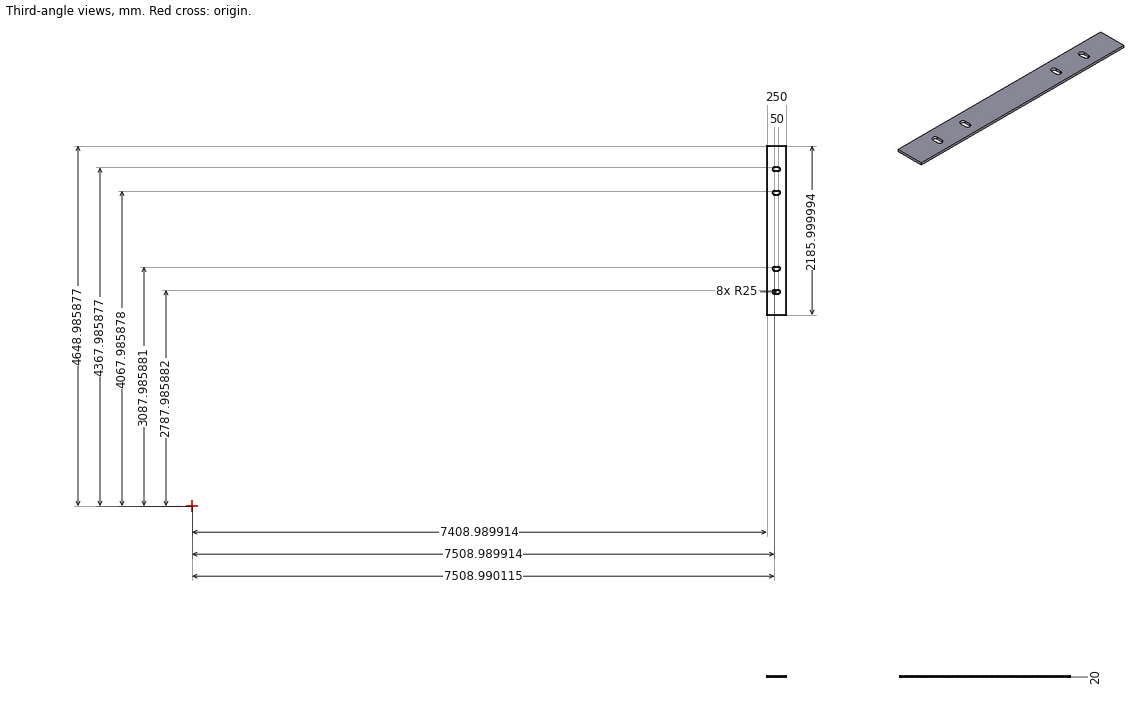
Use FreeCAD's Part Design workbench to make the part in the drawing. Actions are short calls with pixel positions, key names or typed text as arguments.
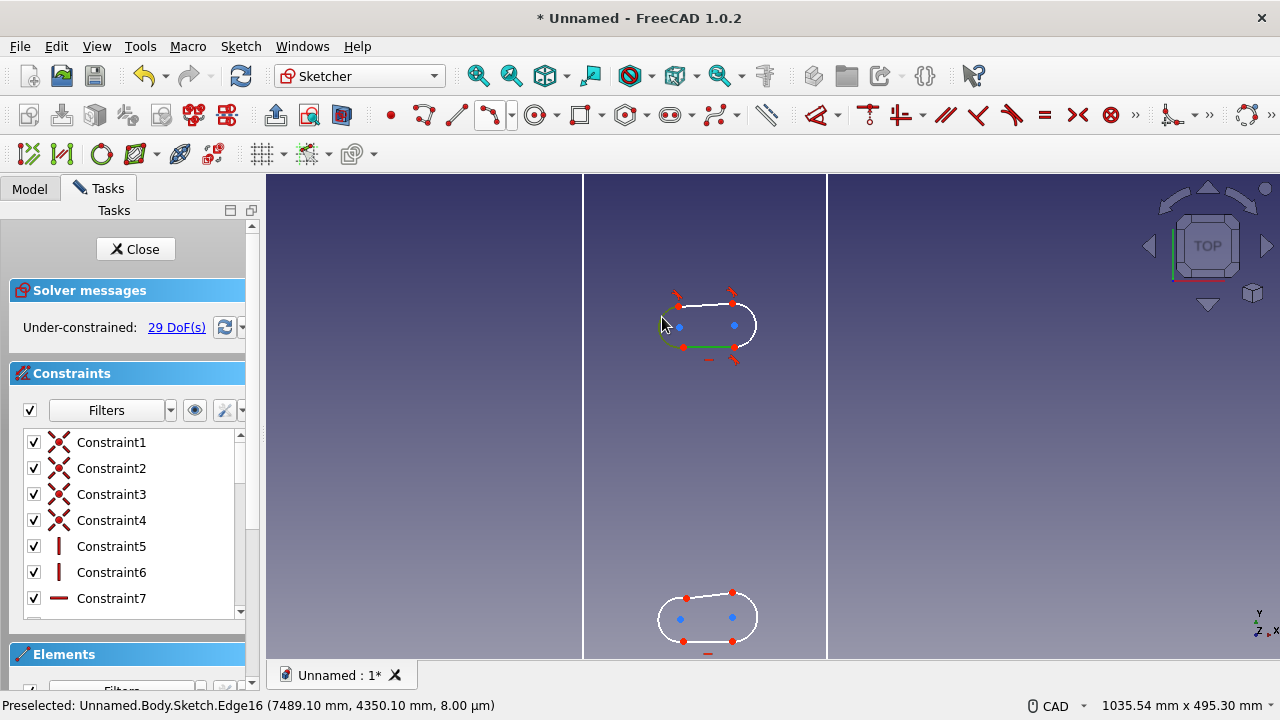
key(t)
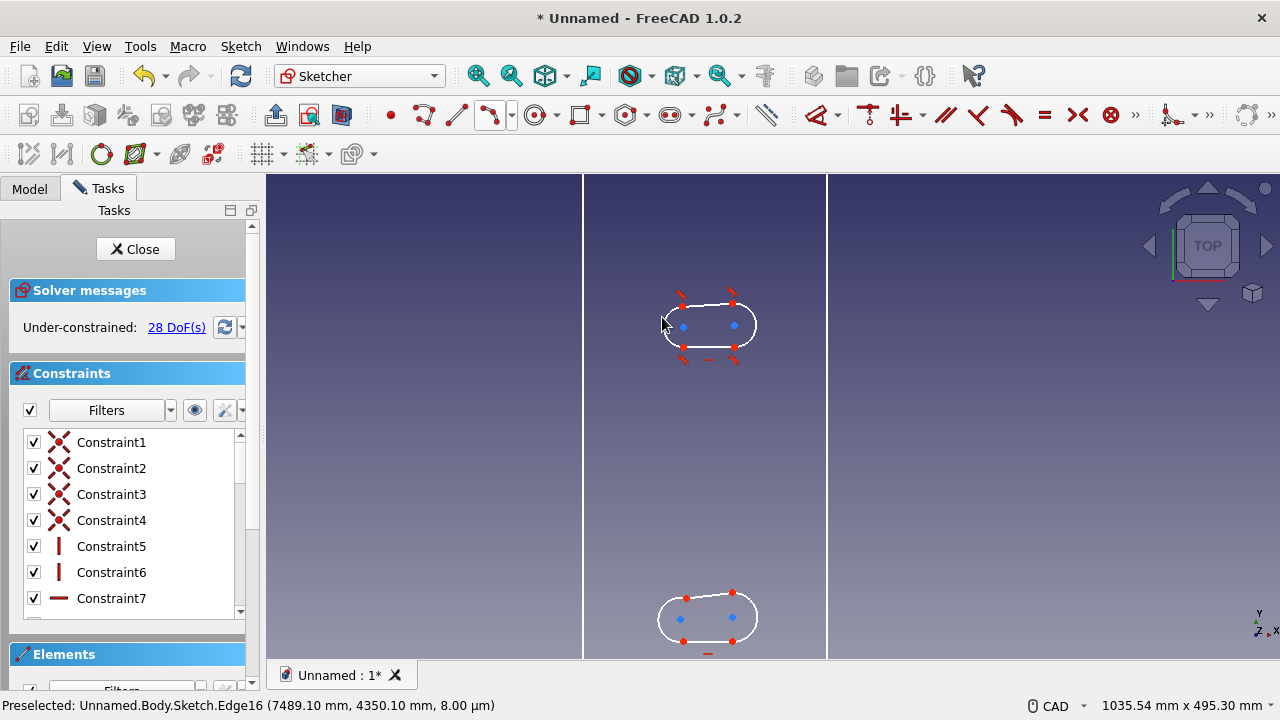
click(700, 597)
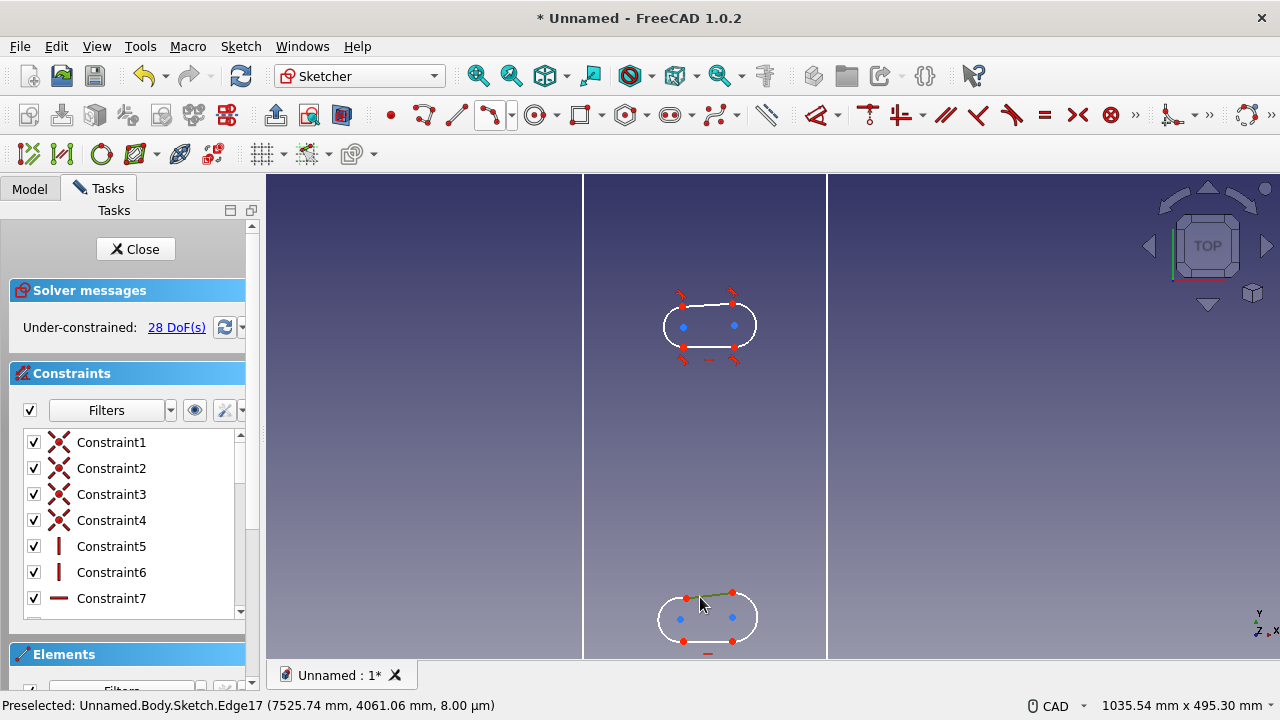
click(753, 603)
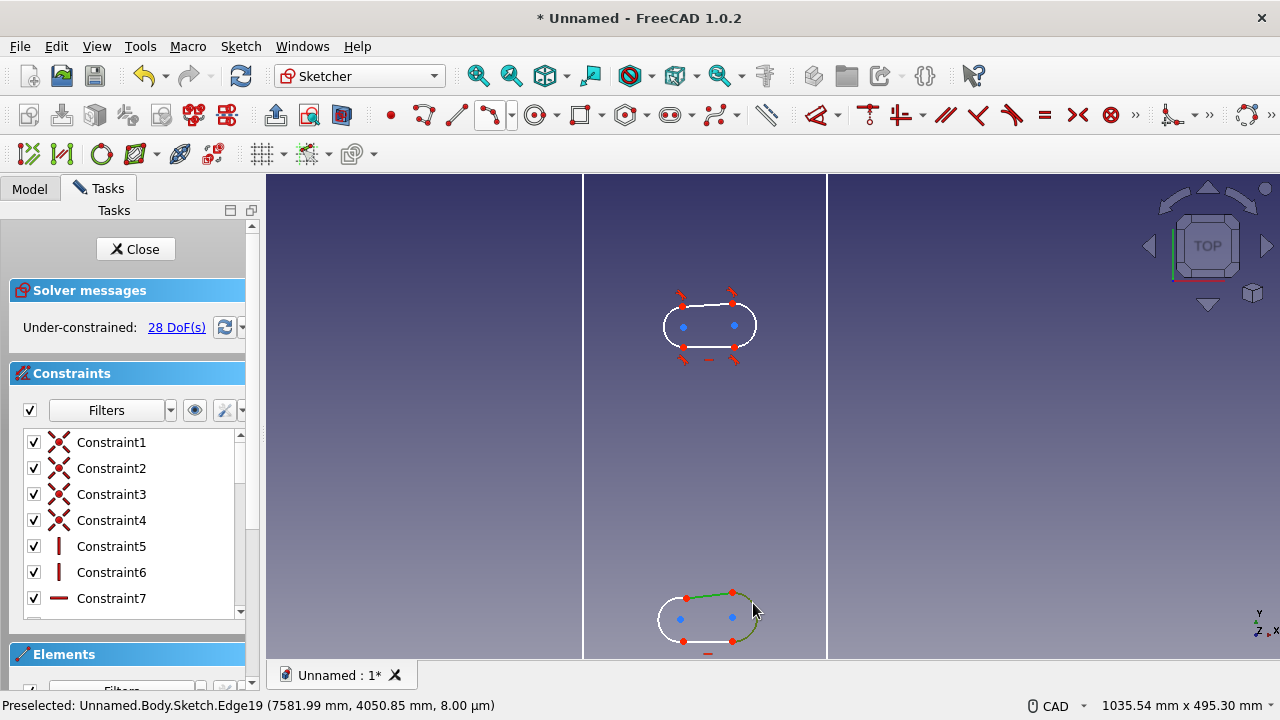
key(t)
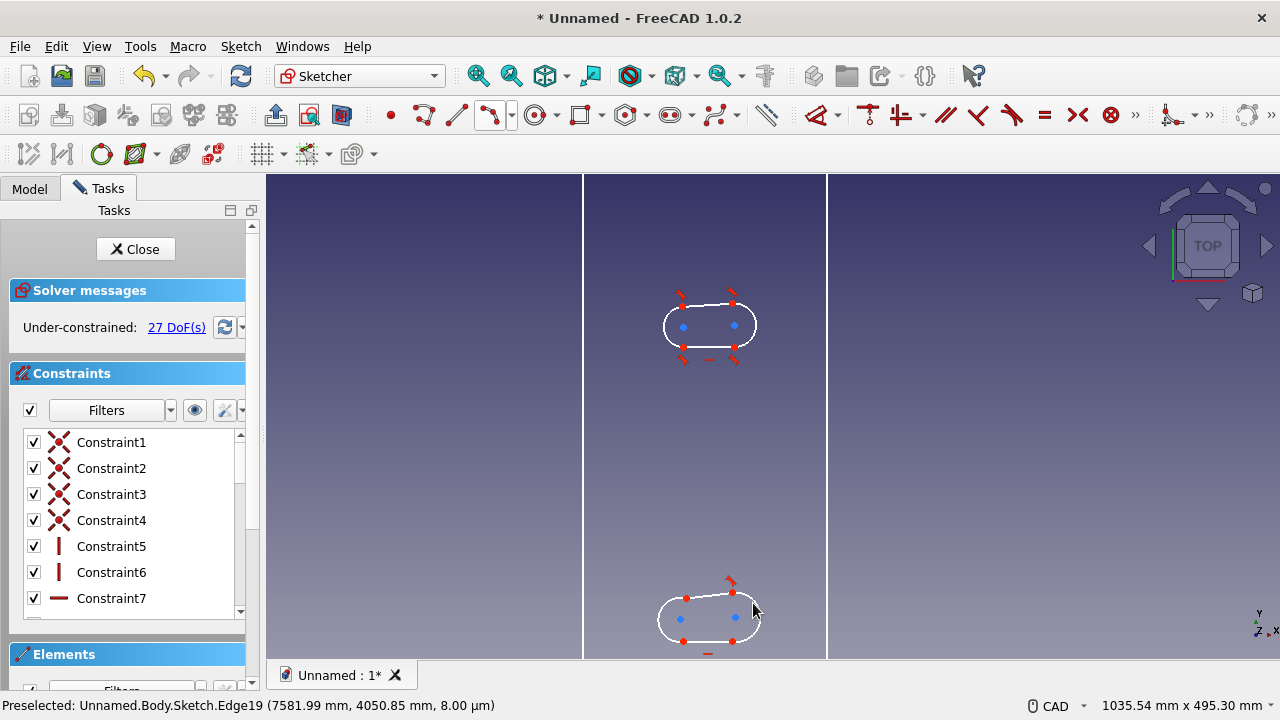
click(700, 597)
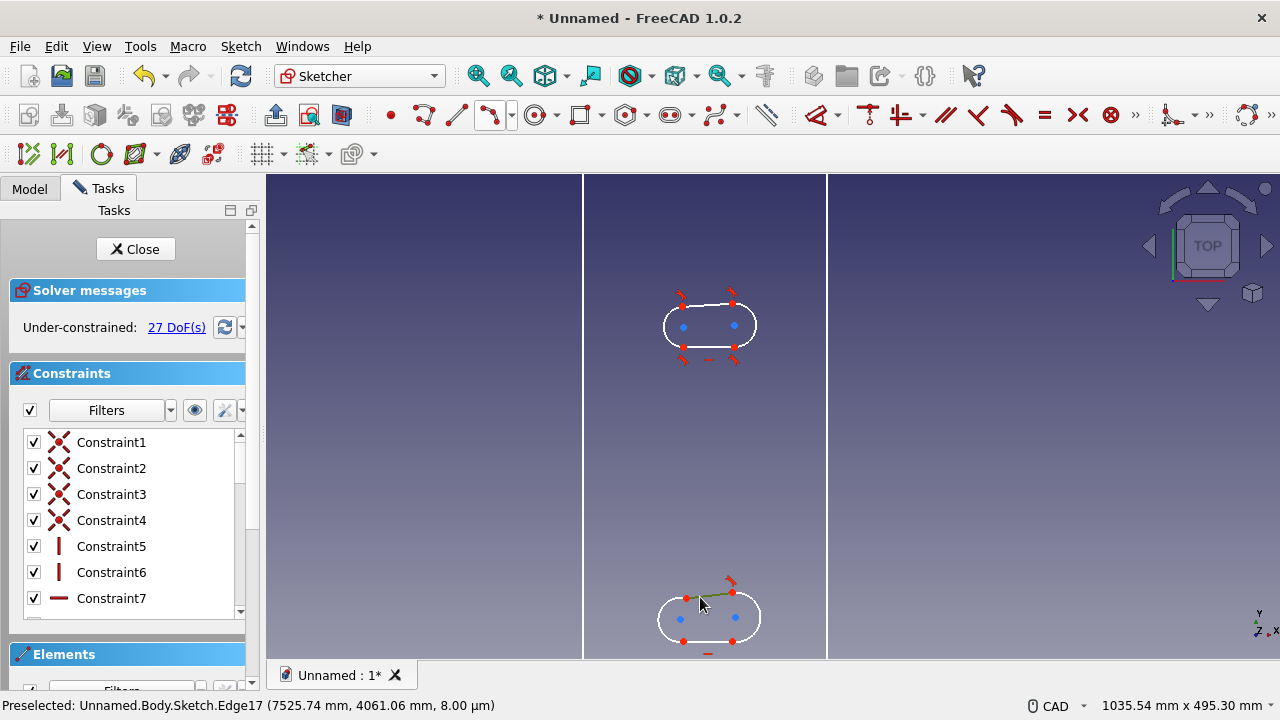
click(665, 604)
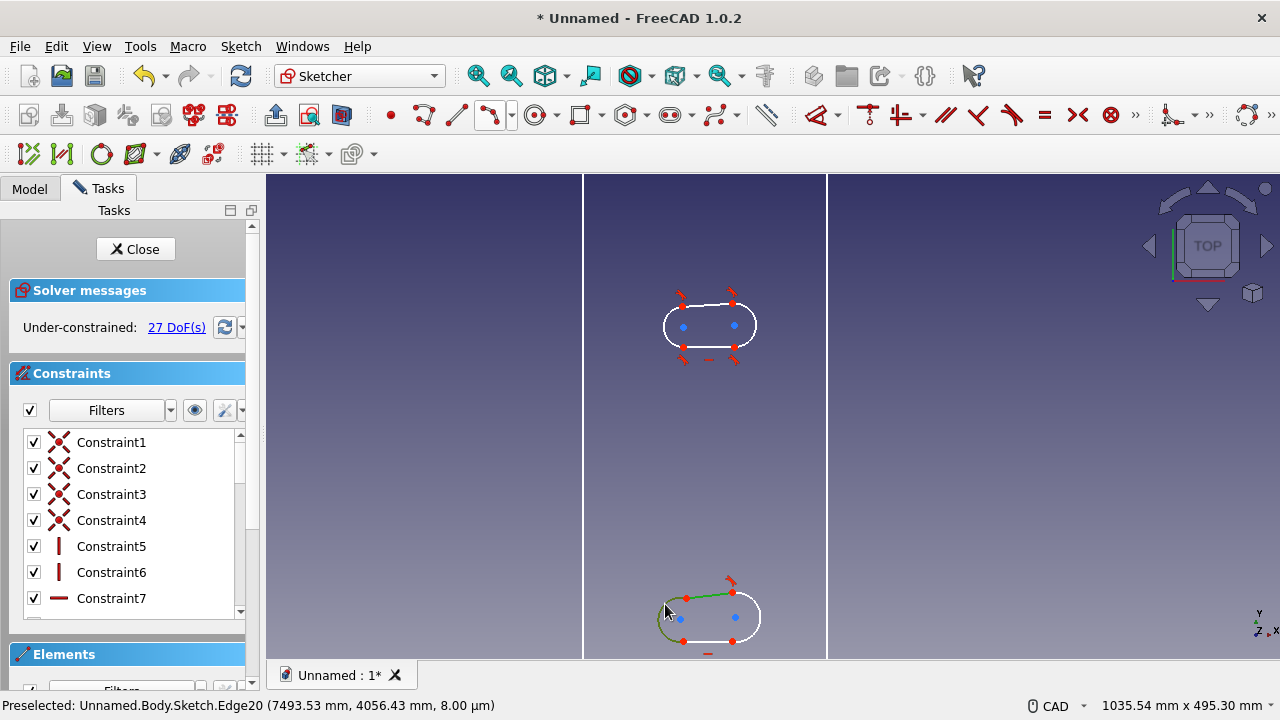
click(1012, 116)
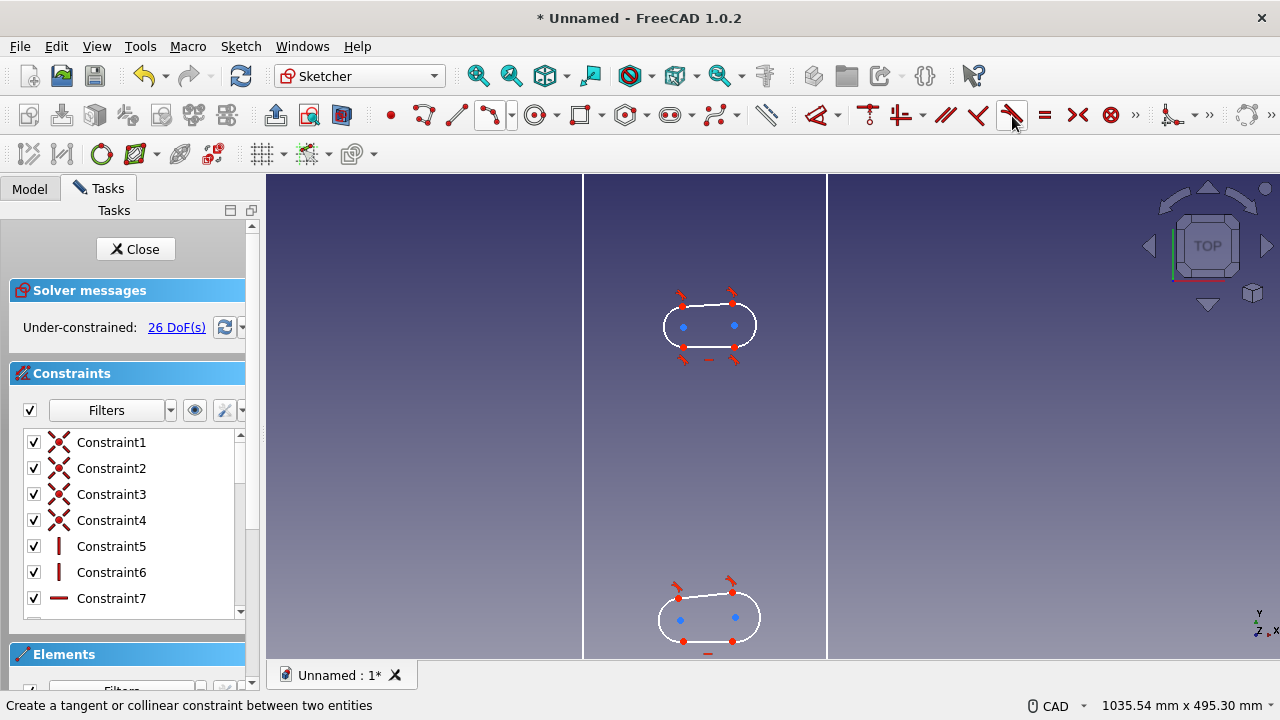
scroll(704, 311, down, 10)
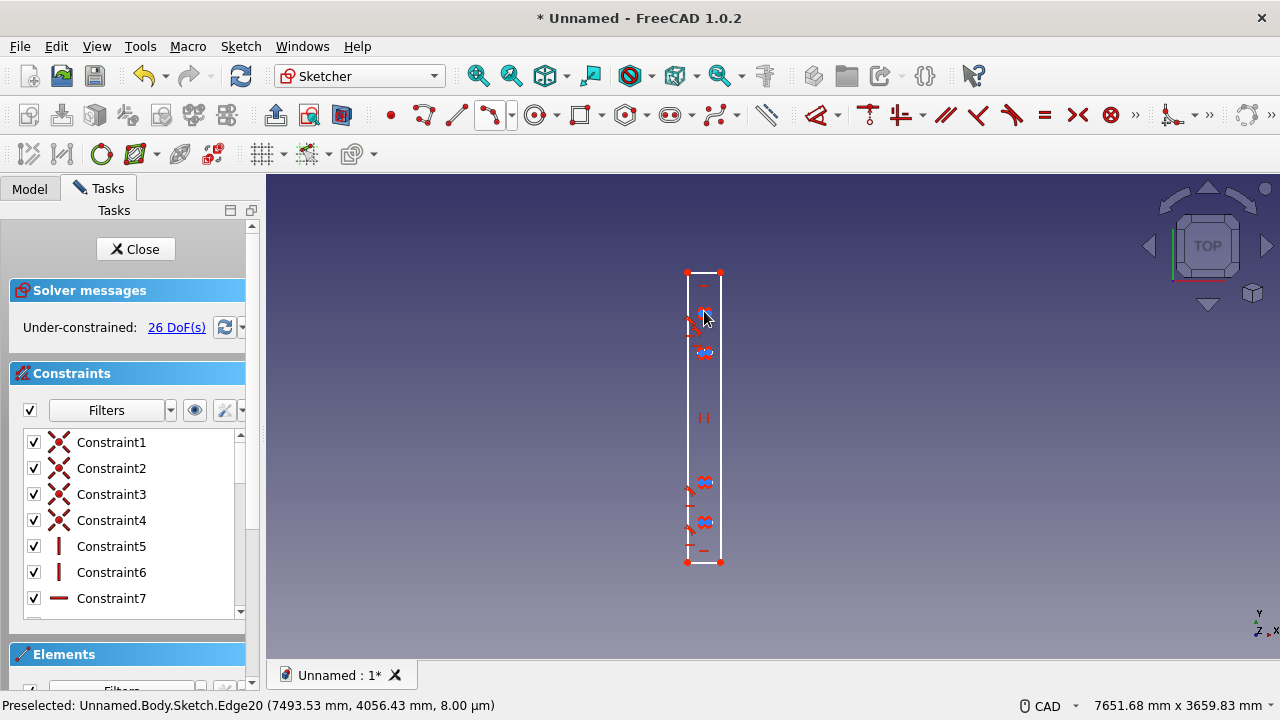
scroll(706, 356, up, 10)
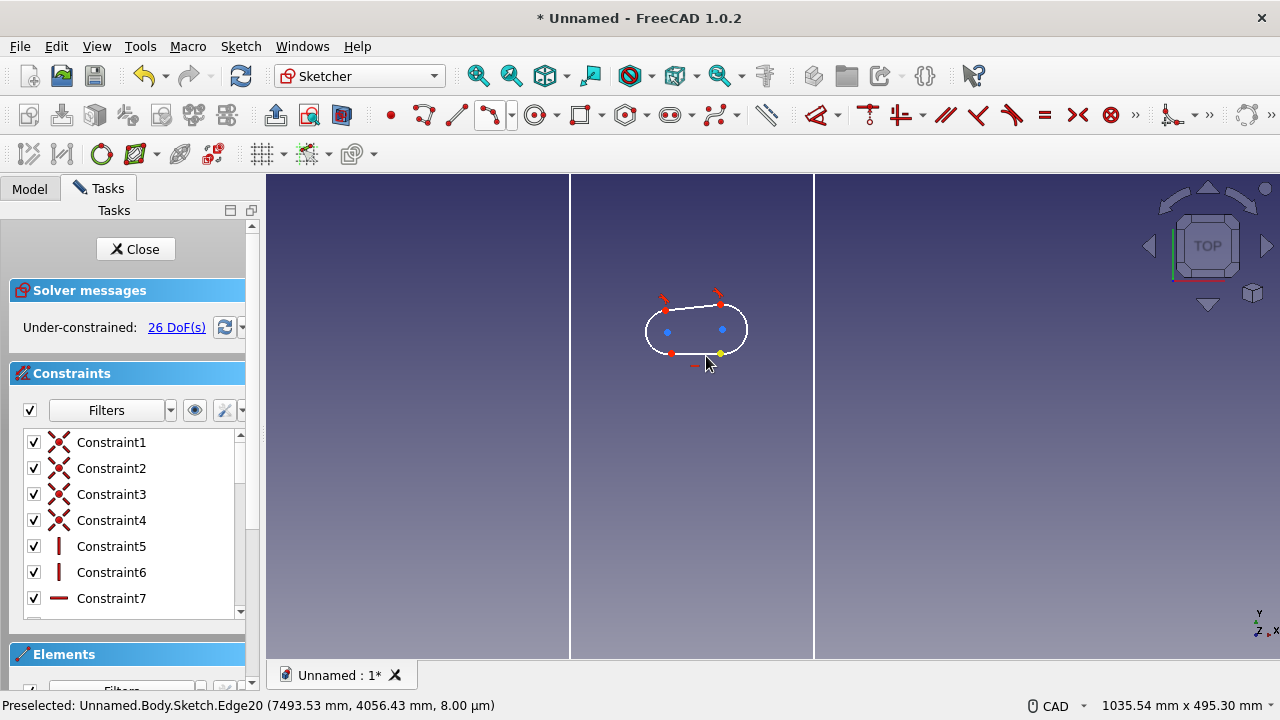
click(705, 354)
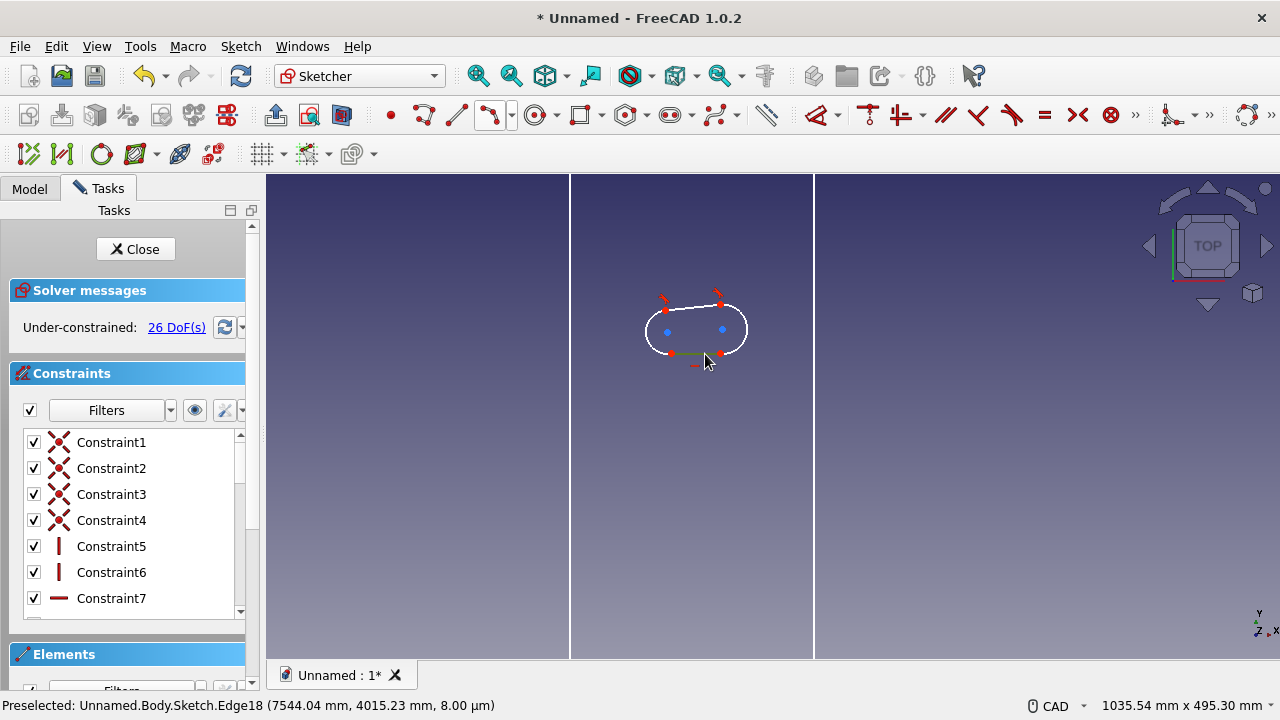
click(742, 345)